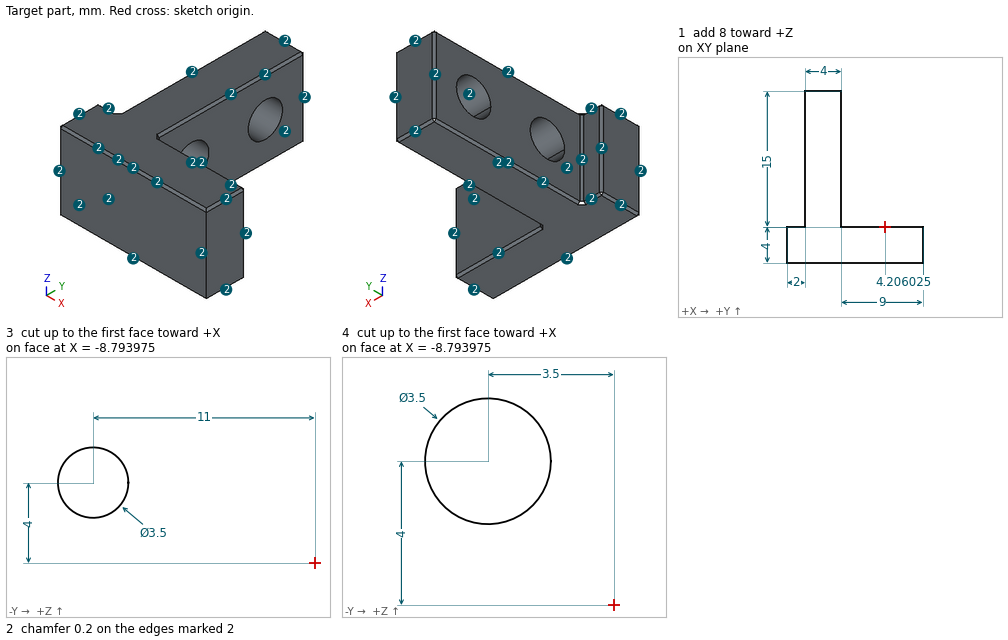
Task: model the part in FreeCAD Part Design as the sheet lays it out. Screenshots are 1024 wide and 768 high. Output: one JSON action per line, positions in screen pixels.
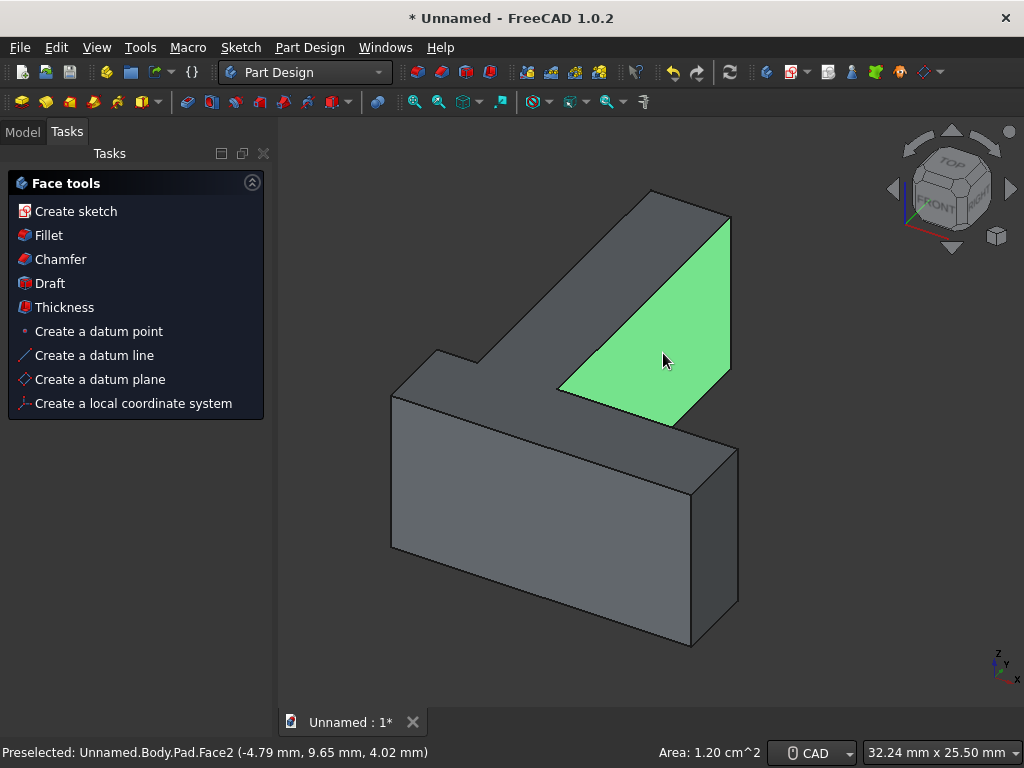
{"action": "left_click", "coordinate": [643, 457], "text": "ctrl"}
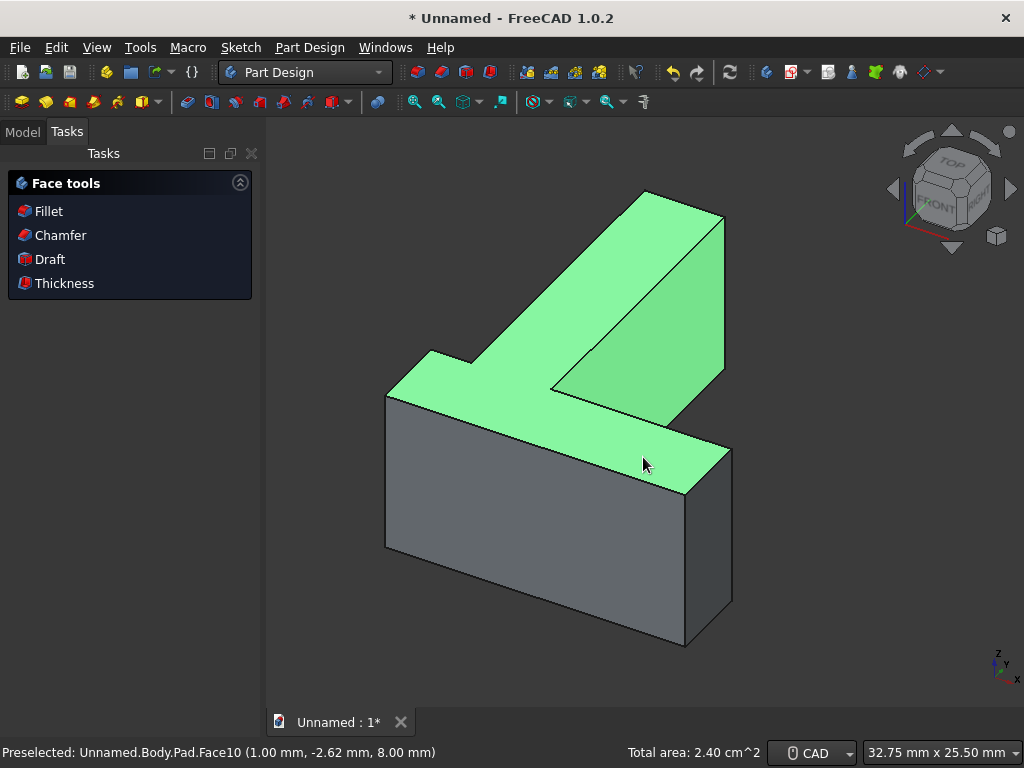
{"action": "key", "text": "0"}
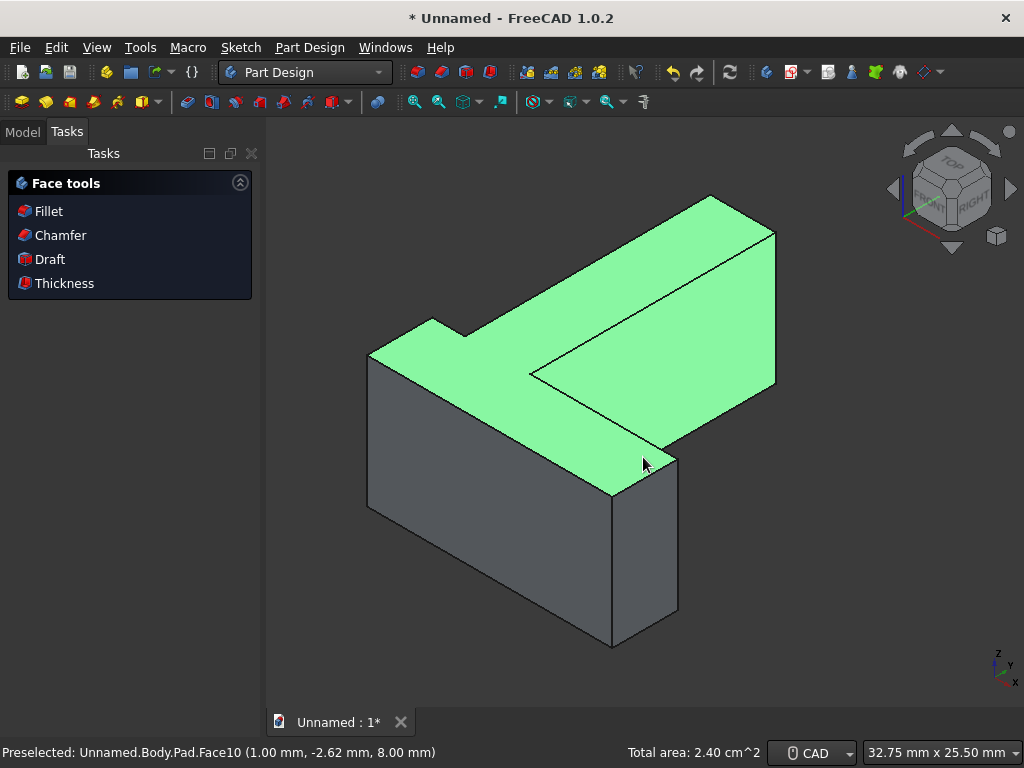
{"action": "key", "text": "2"}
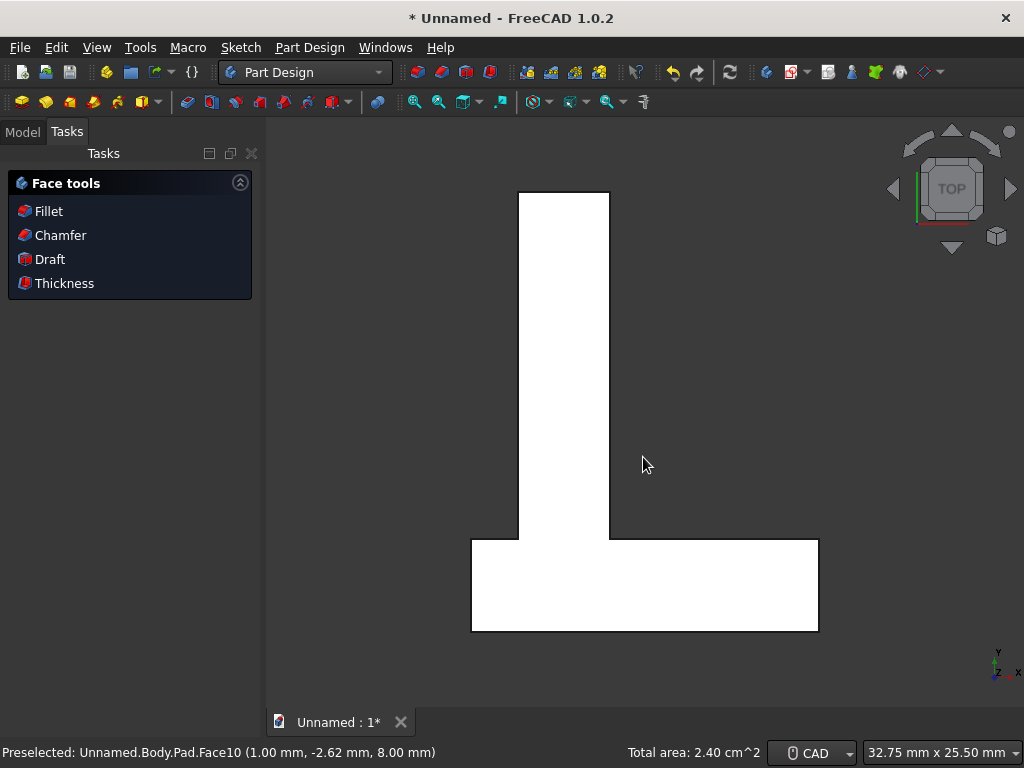
{"action": "key", "text": "1"}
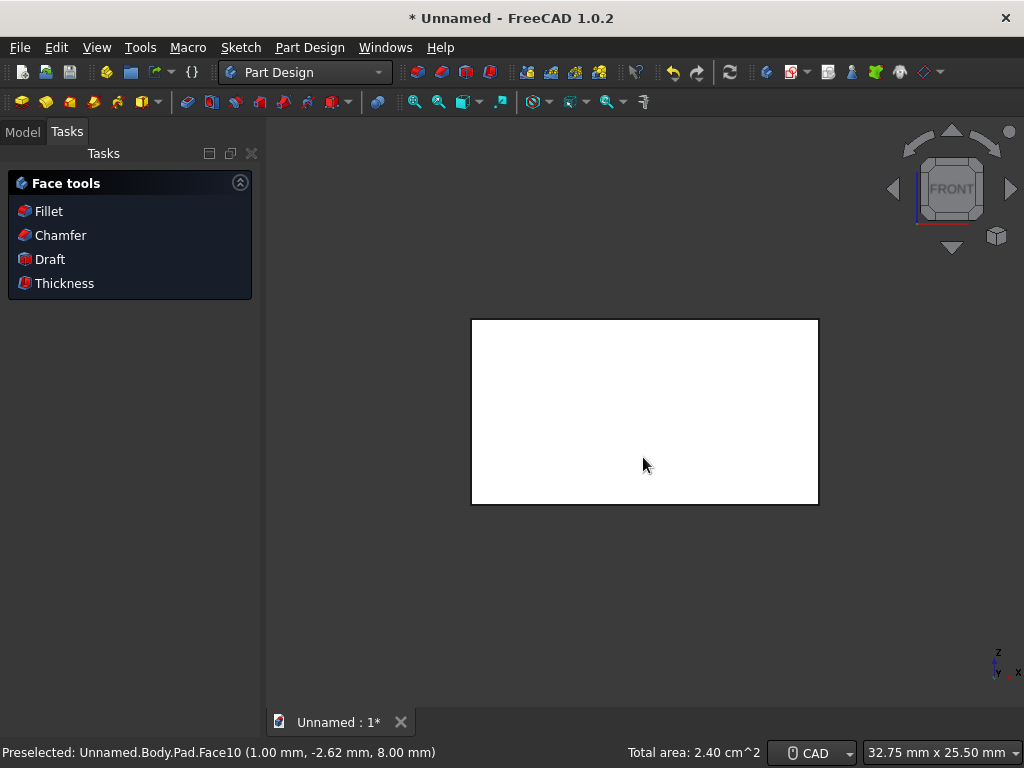
{"action": "left_click", "coordinate": [471, 411], "text": "ctrl"}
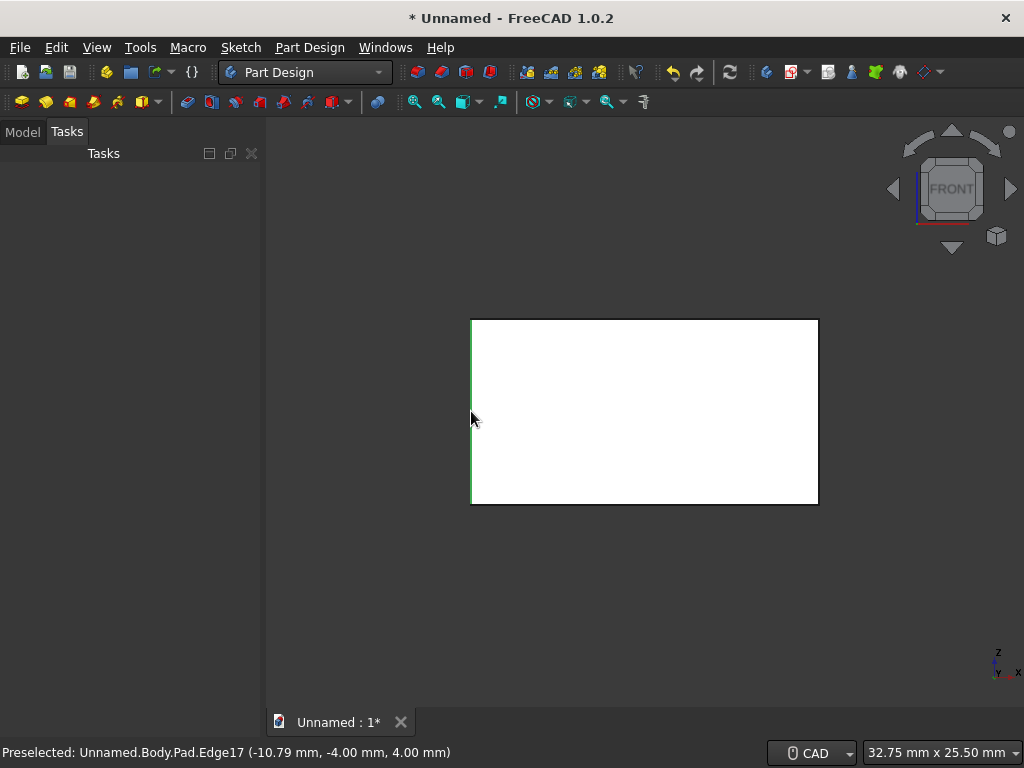
{"action": "key", "text": "3"}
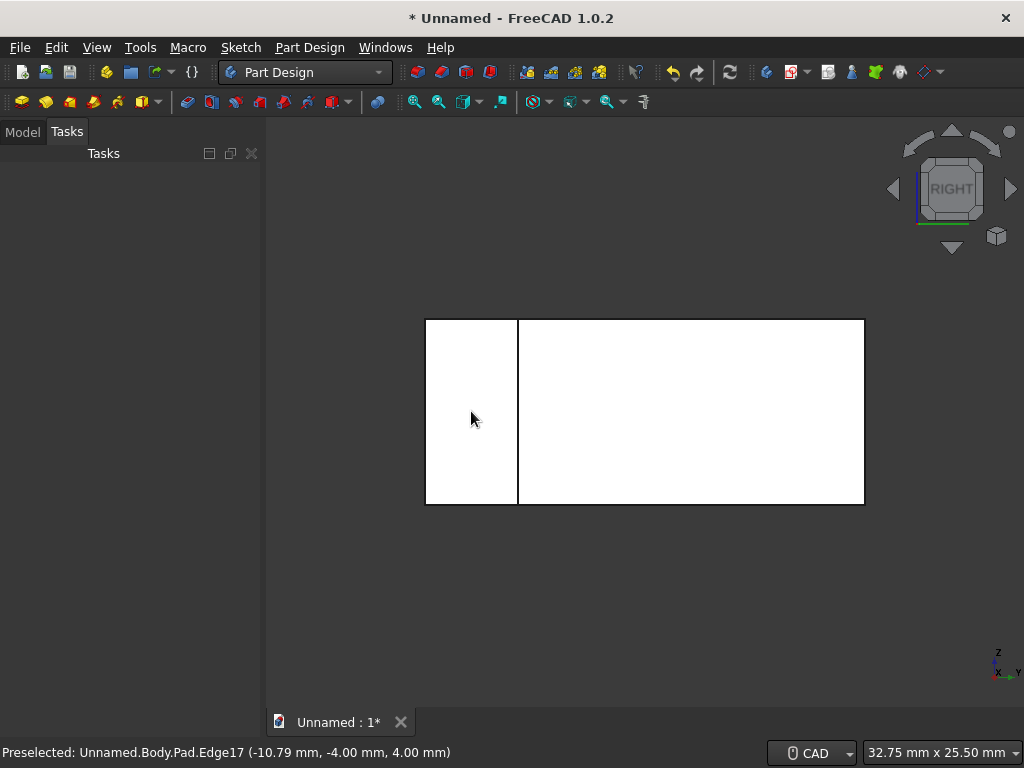
{"action": "left_click", "coordinate": [518, 411], "text": "ctrl"}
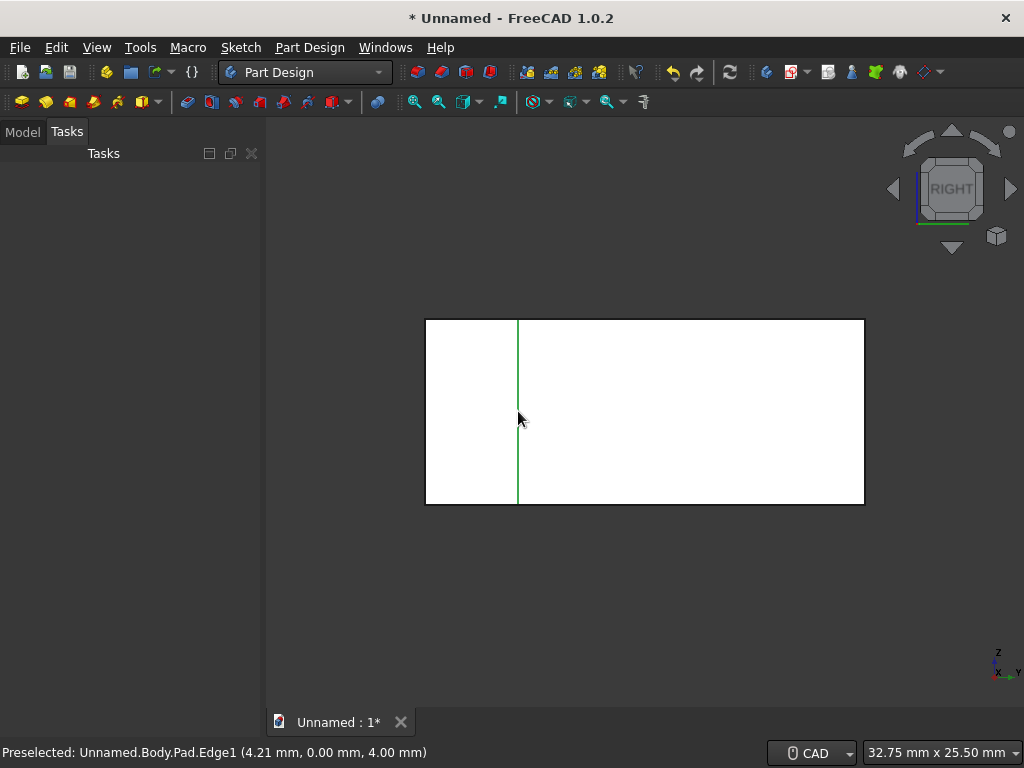
{"action": "key", "text": "5"}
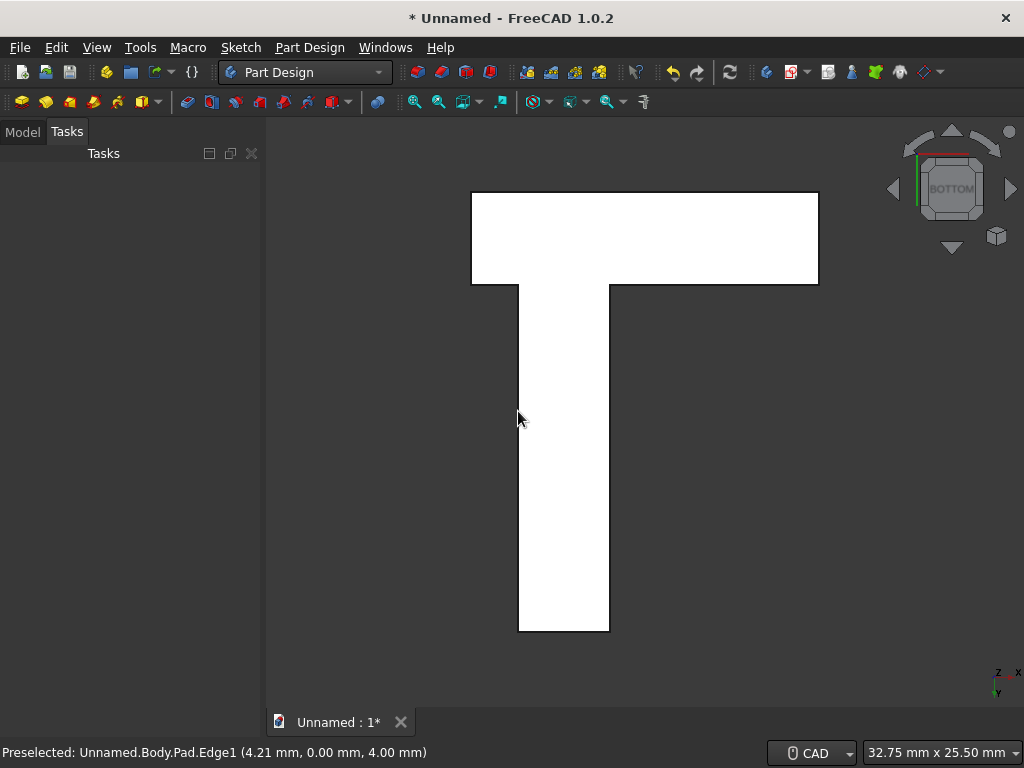
{"action": "left_click", "coordinate": [744, 223], "text": "ctrl"}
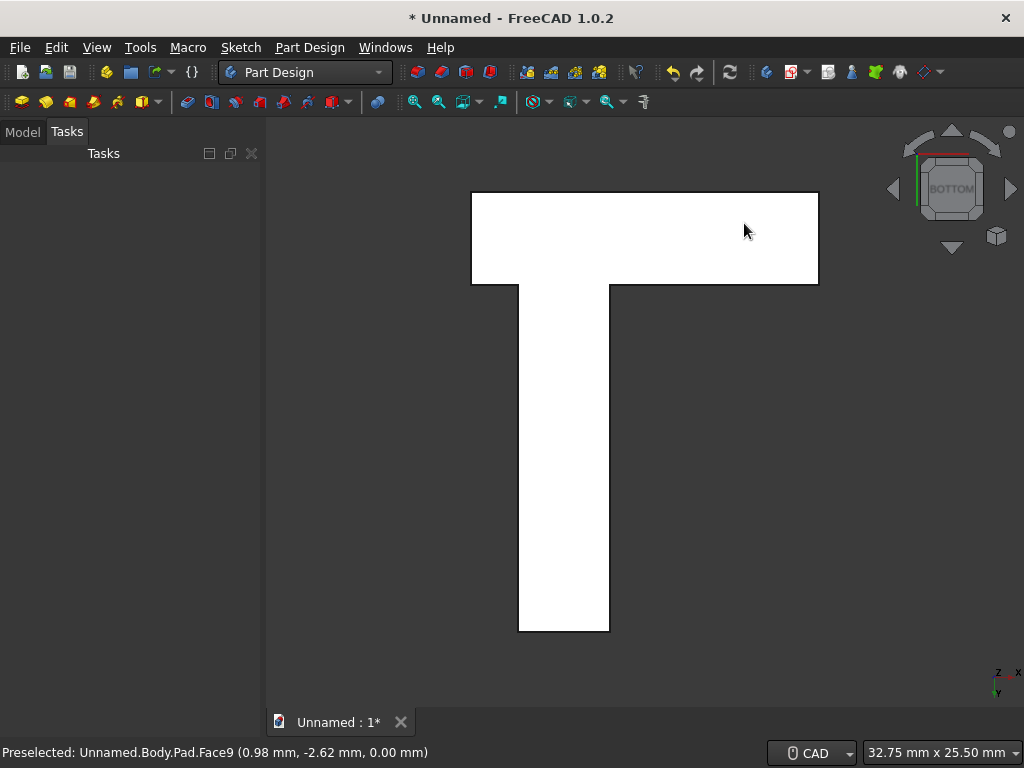
{"action": "key", "text": "4"}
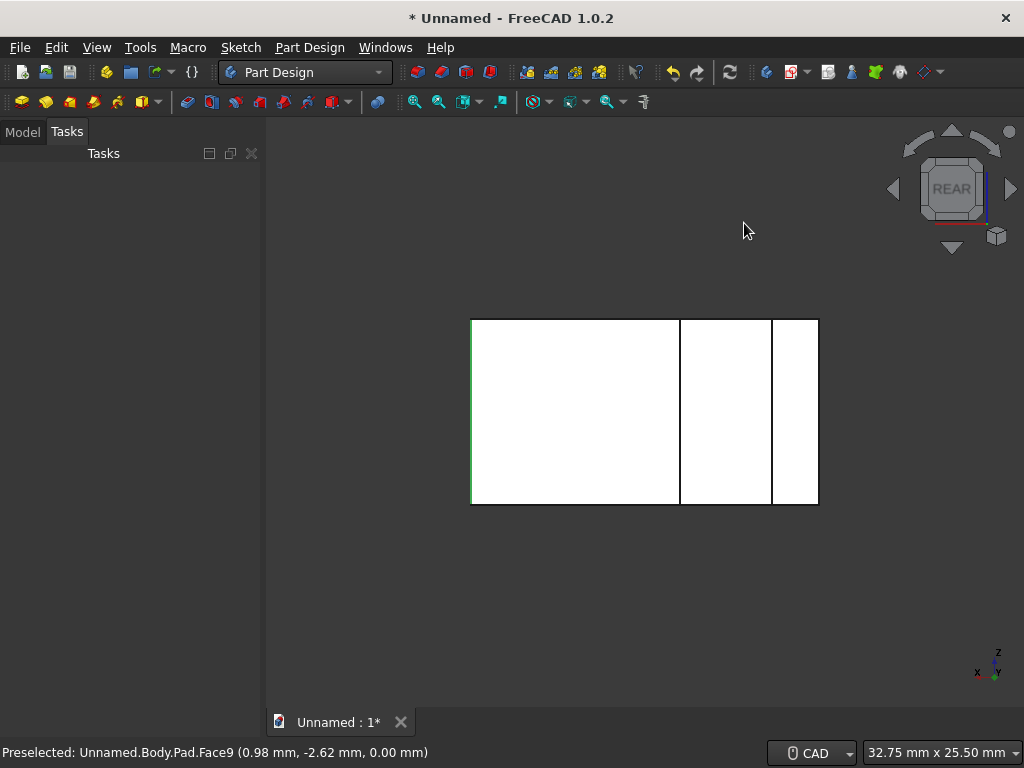
{"action": "left_click", "coordinate": [819, 411], "text": "ctrl"}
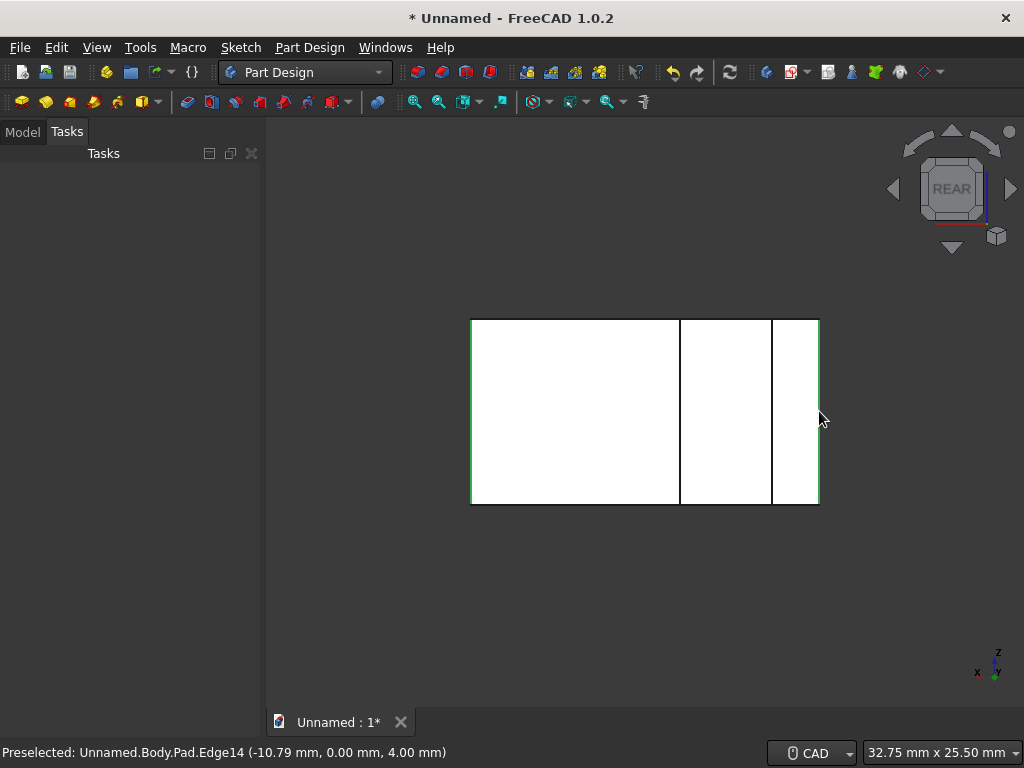
{"action": "key", "text": "6"}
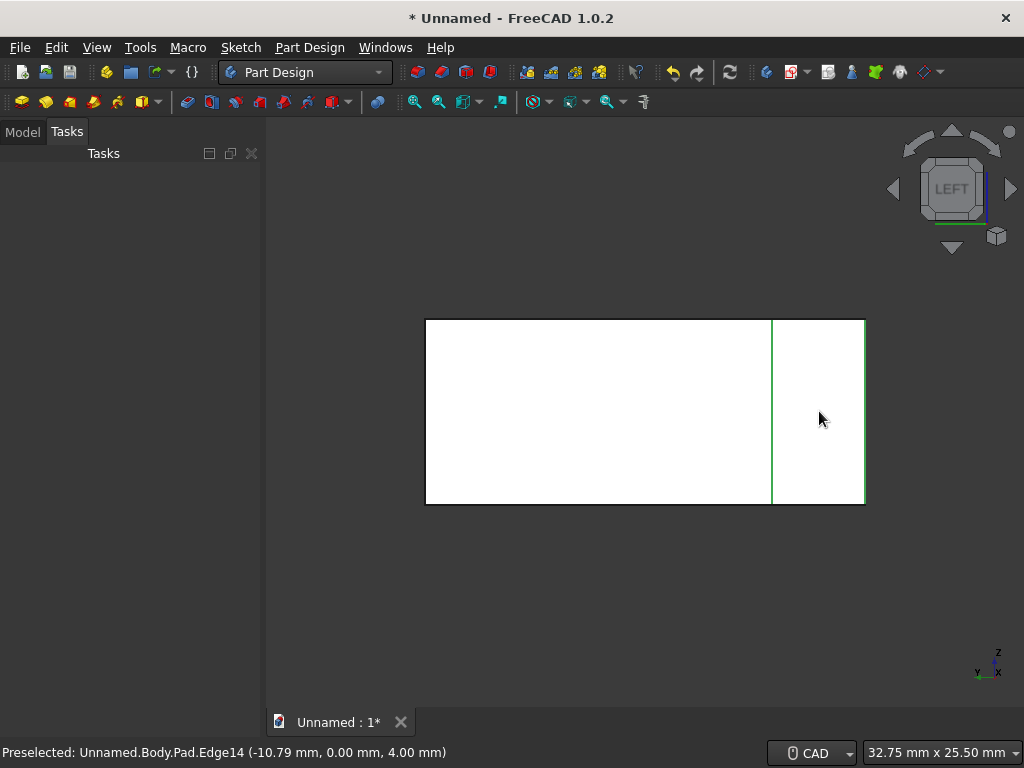
{"action": "left_click", "coordinate": [549, 411], "text": "ctrl"}